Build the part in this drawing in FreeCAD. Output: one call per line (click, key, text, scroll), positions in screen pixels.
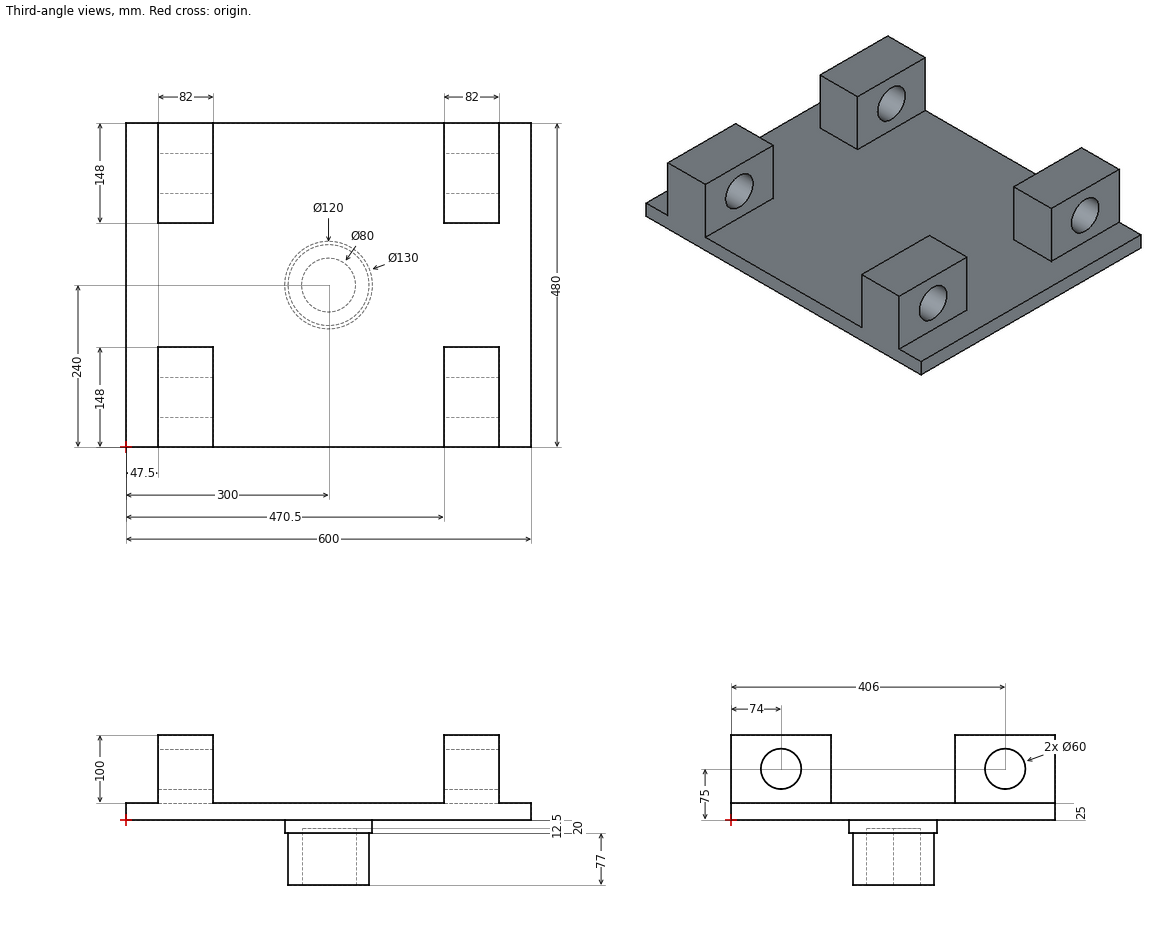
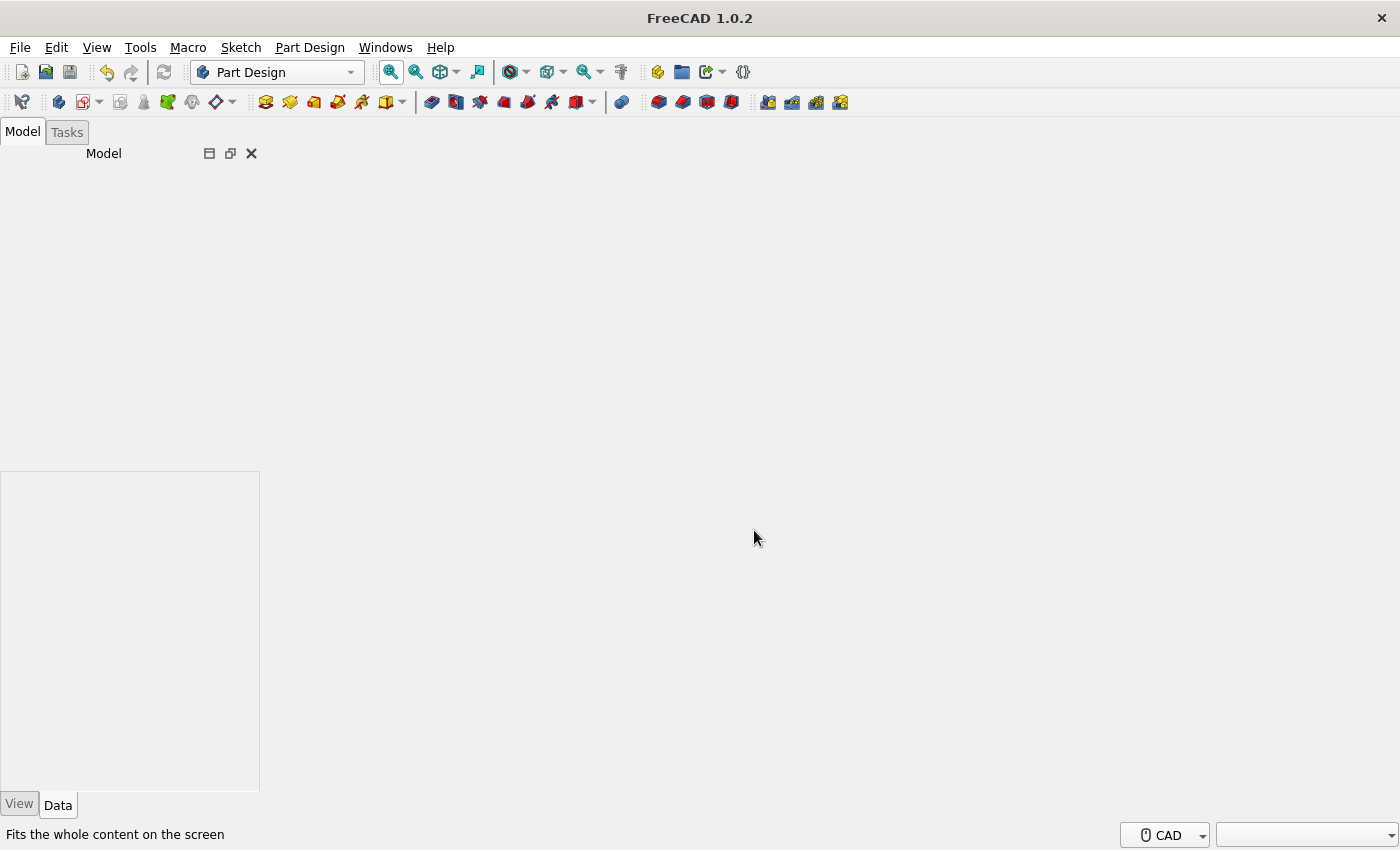
click(22, 72)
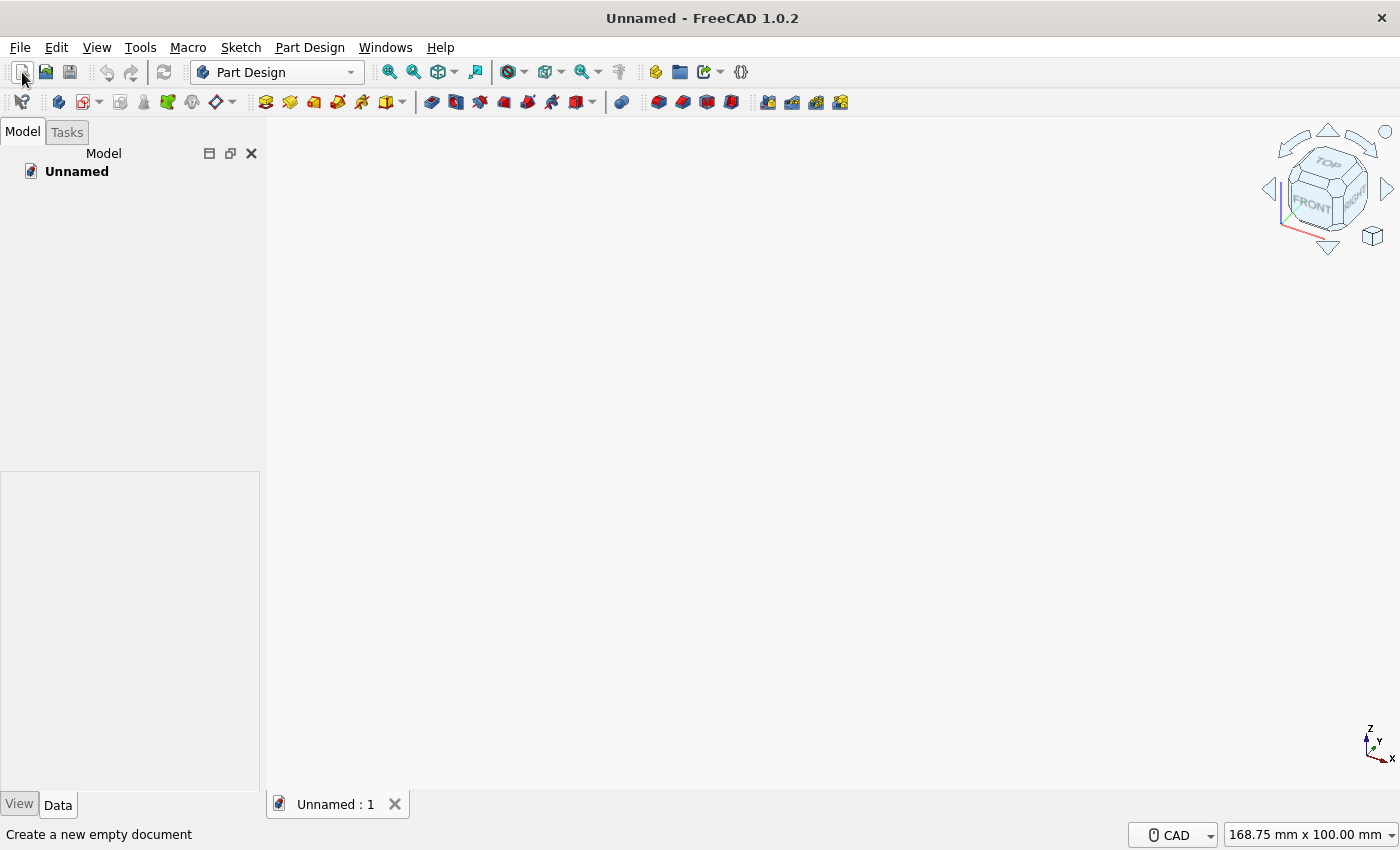
click(84, 102)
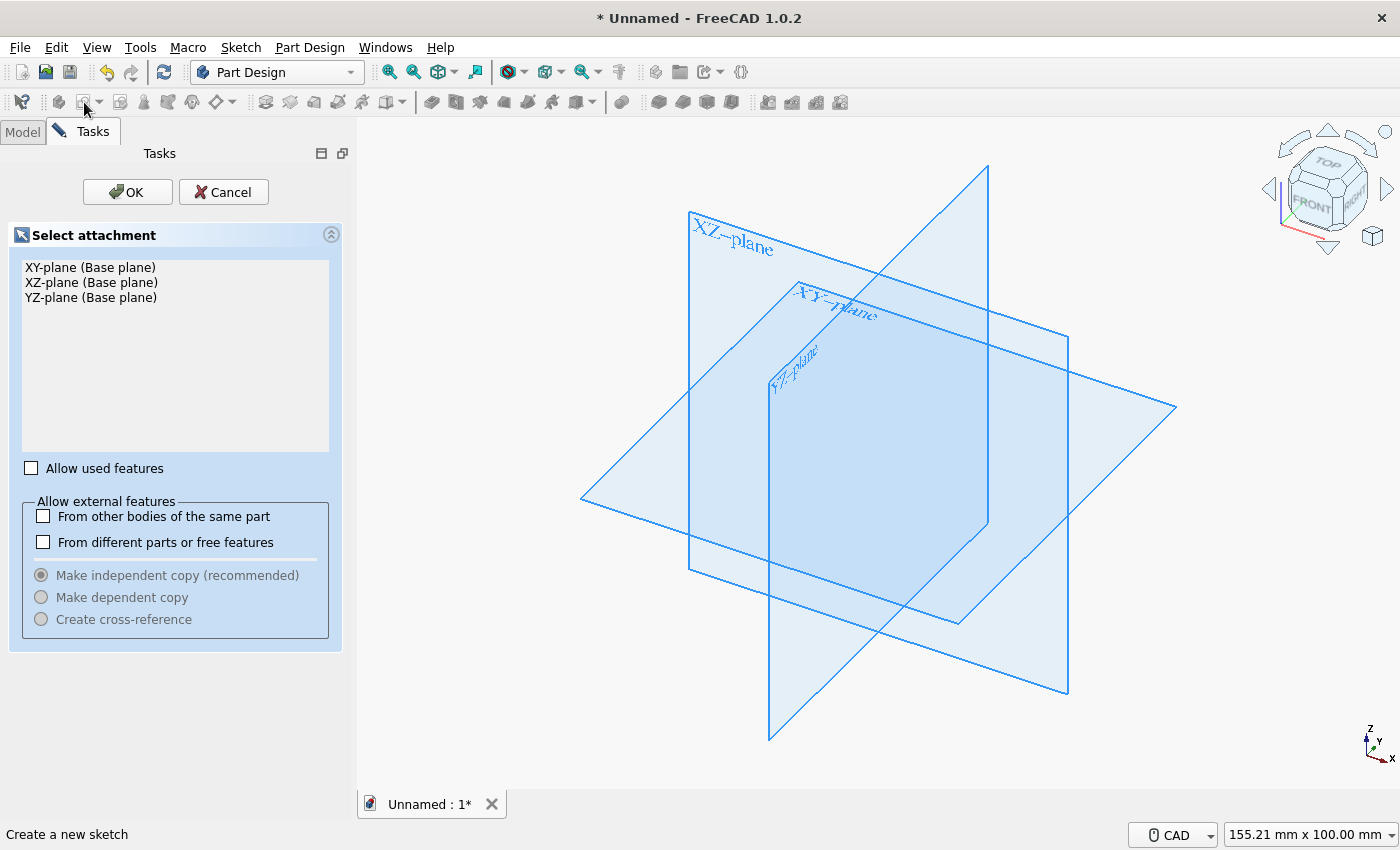
click(82, 268)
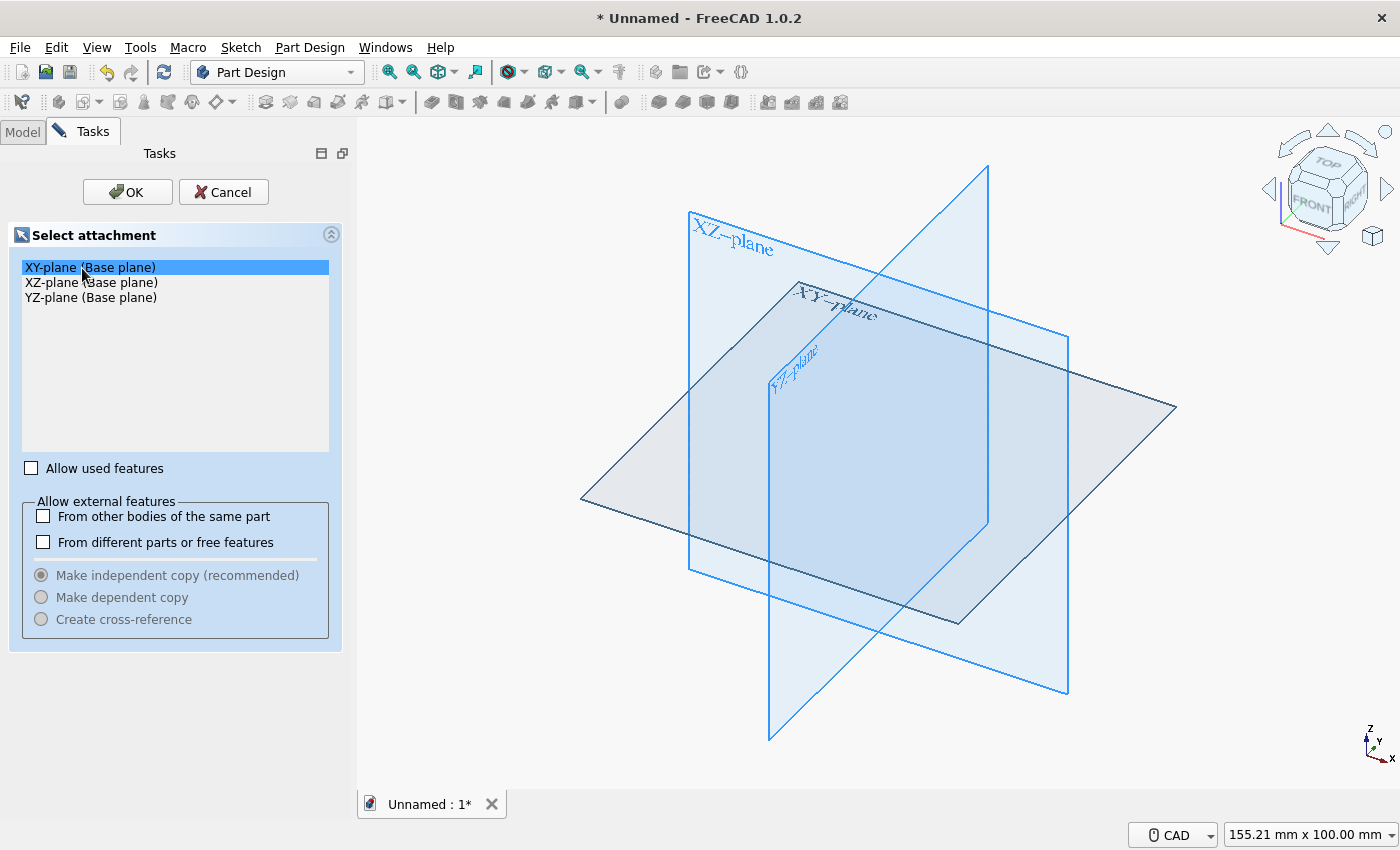
click(128, 192)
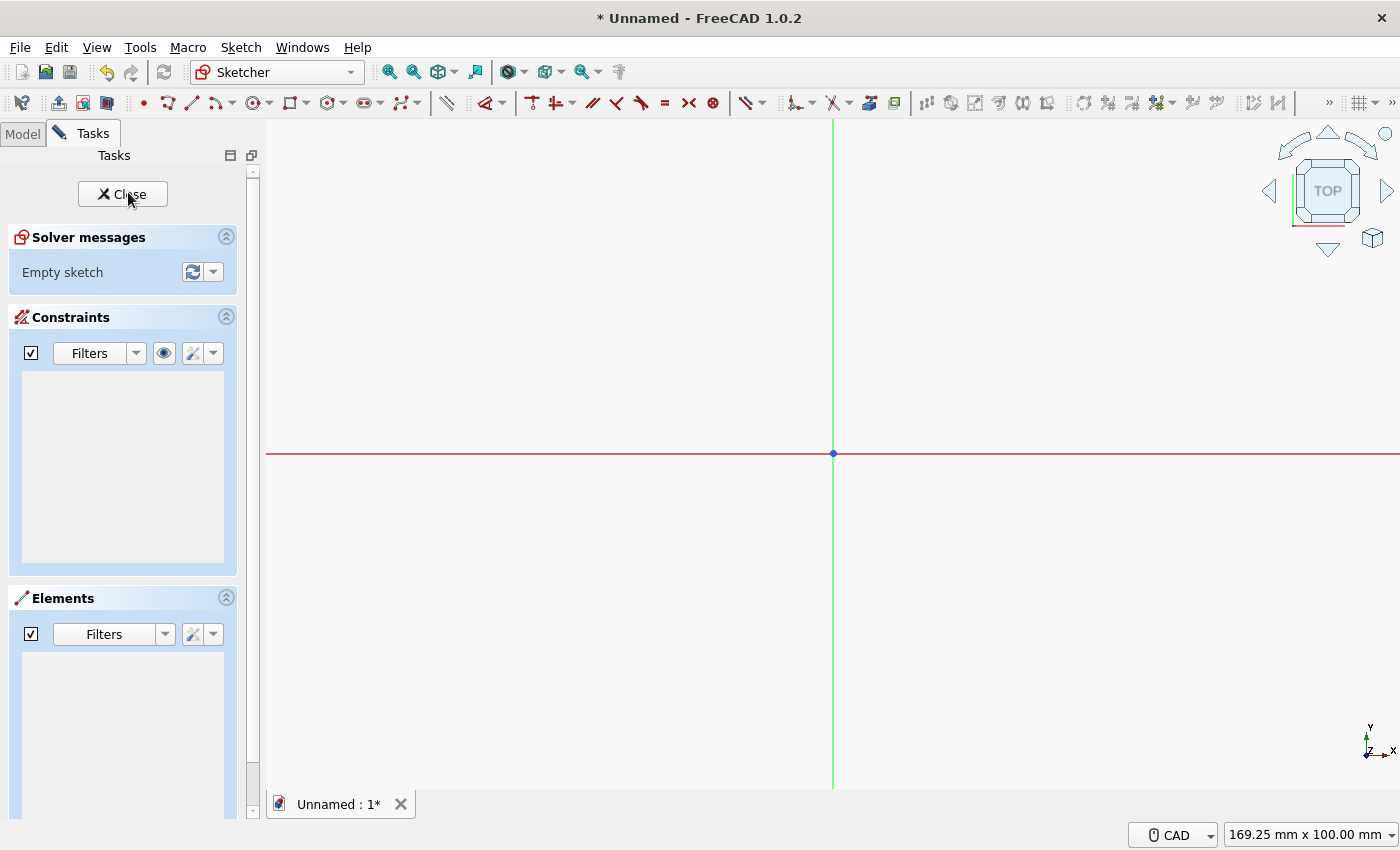
scroll(439, 706, down, 10)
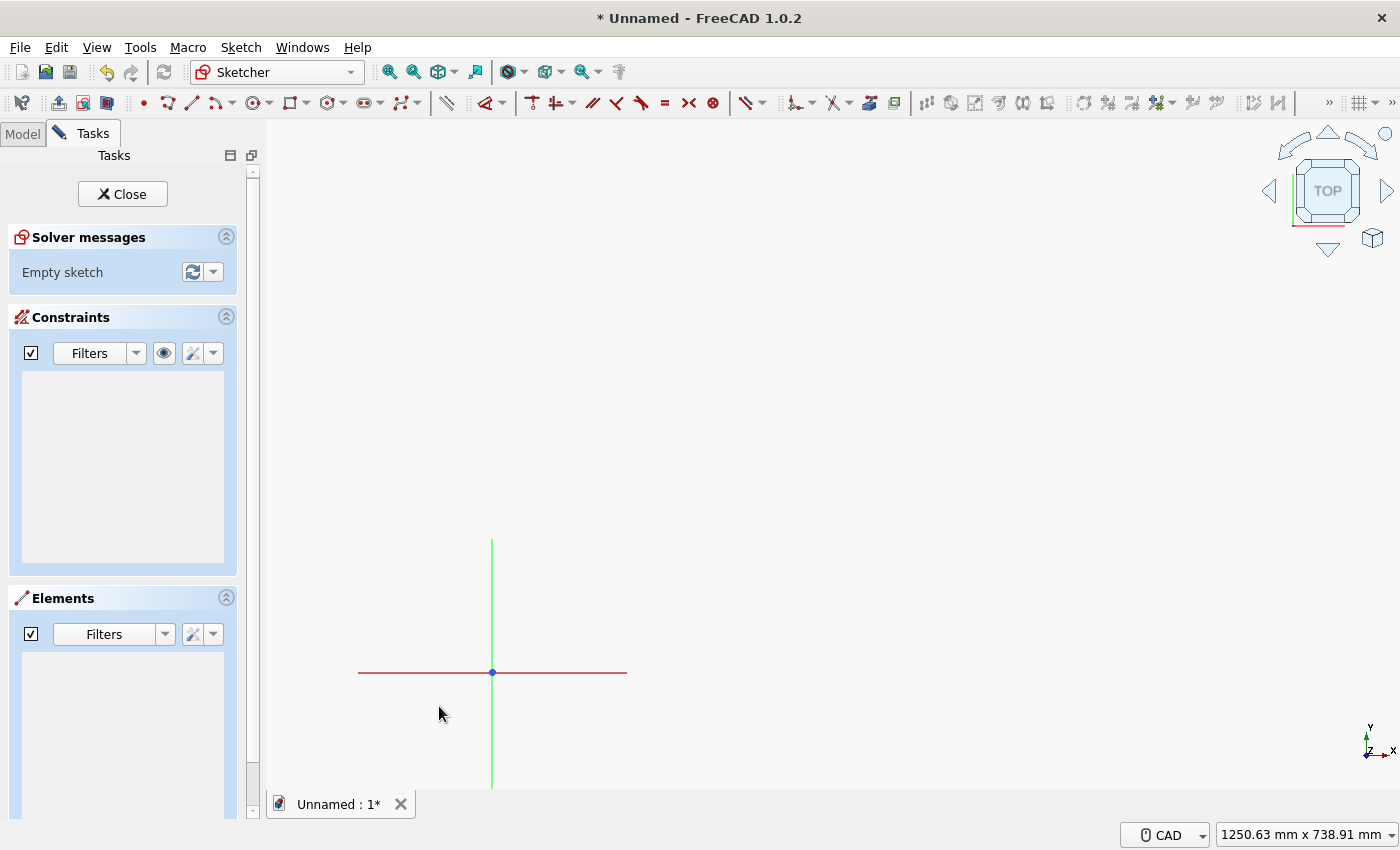
click(290, 104)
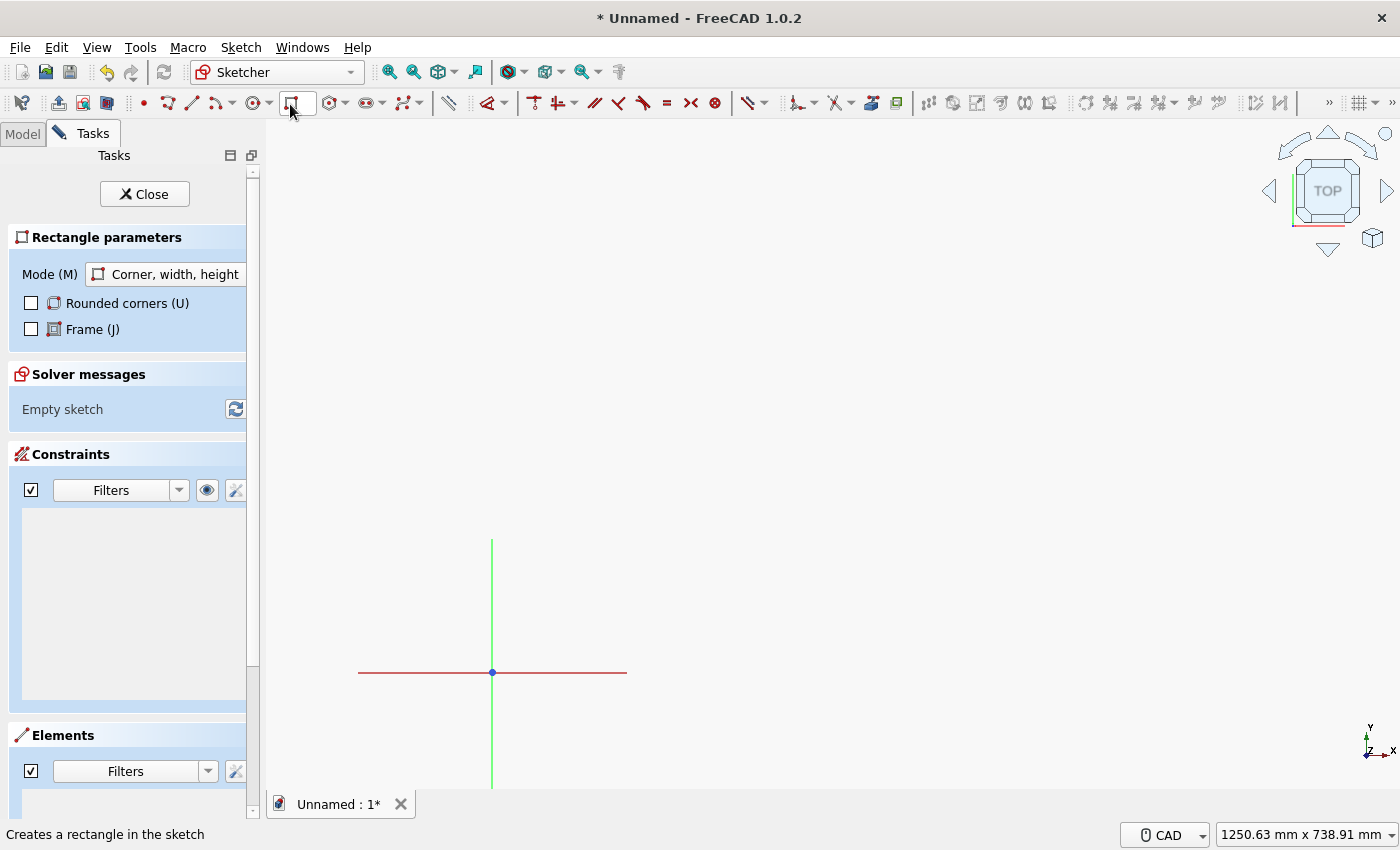
click(492, 673)
move(1037, 237)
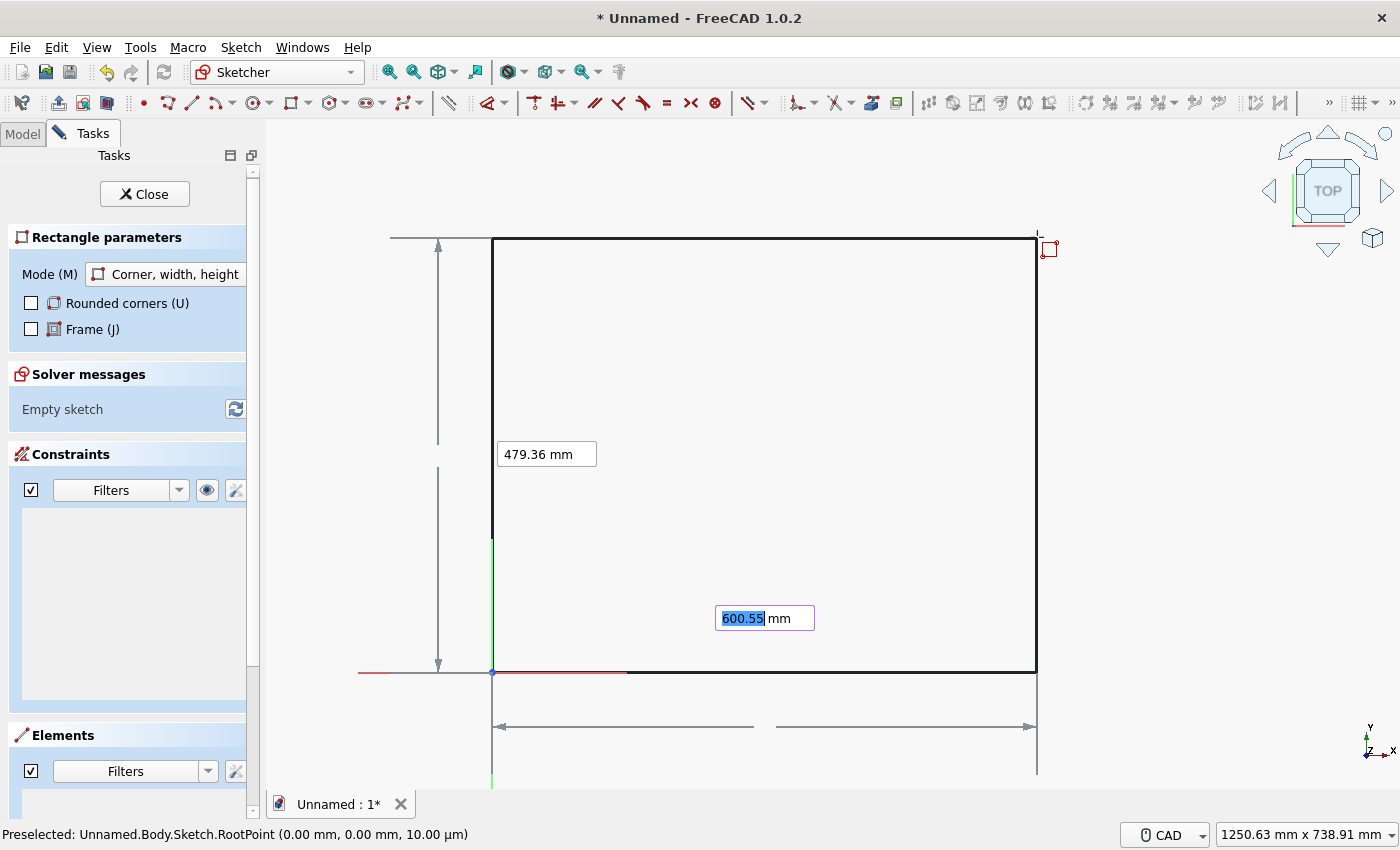
text(600)
key(Tab)
text(480)
key(Return)
key(Escape)